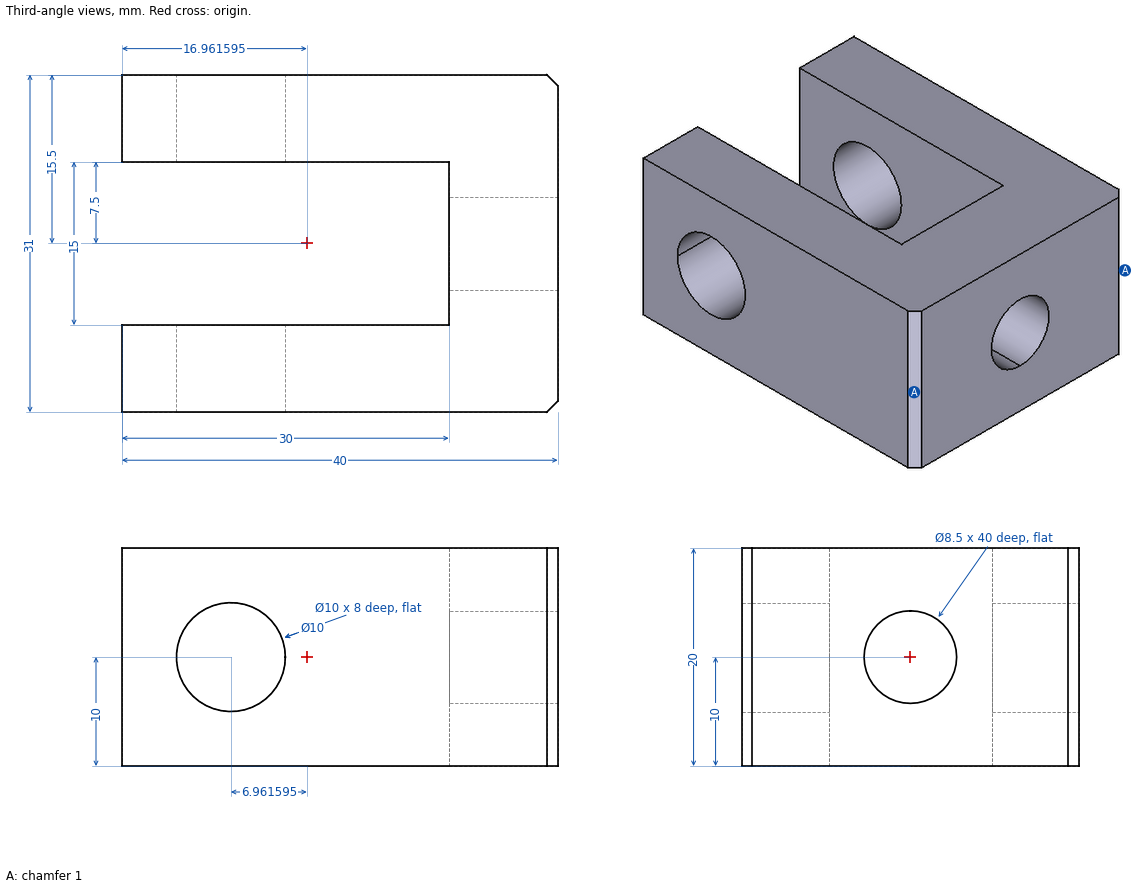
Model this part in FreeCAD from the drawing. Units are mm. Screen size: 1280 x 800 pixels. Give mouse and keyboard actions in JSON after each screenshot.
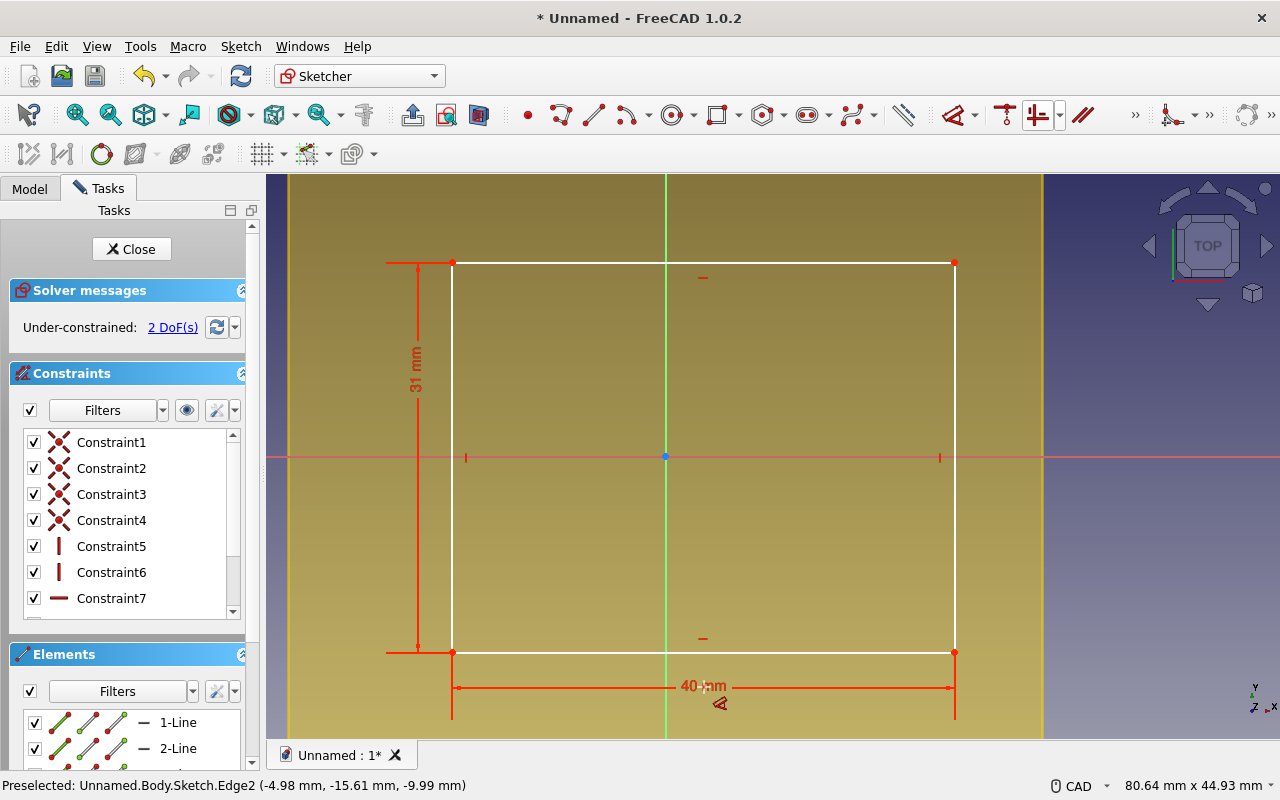
{"action": "left_click", "coordinate": [452, 263]}
{"action": "left_click", "coordinate": [418, 315]}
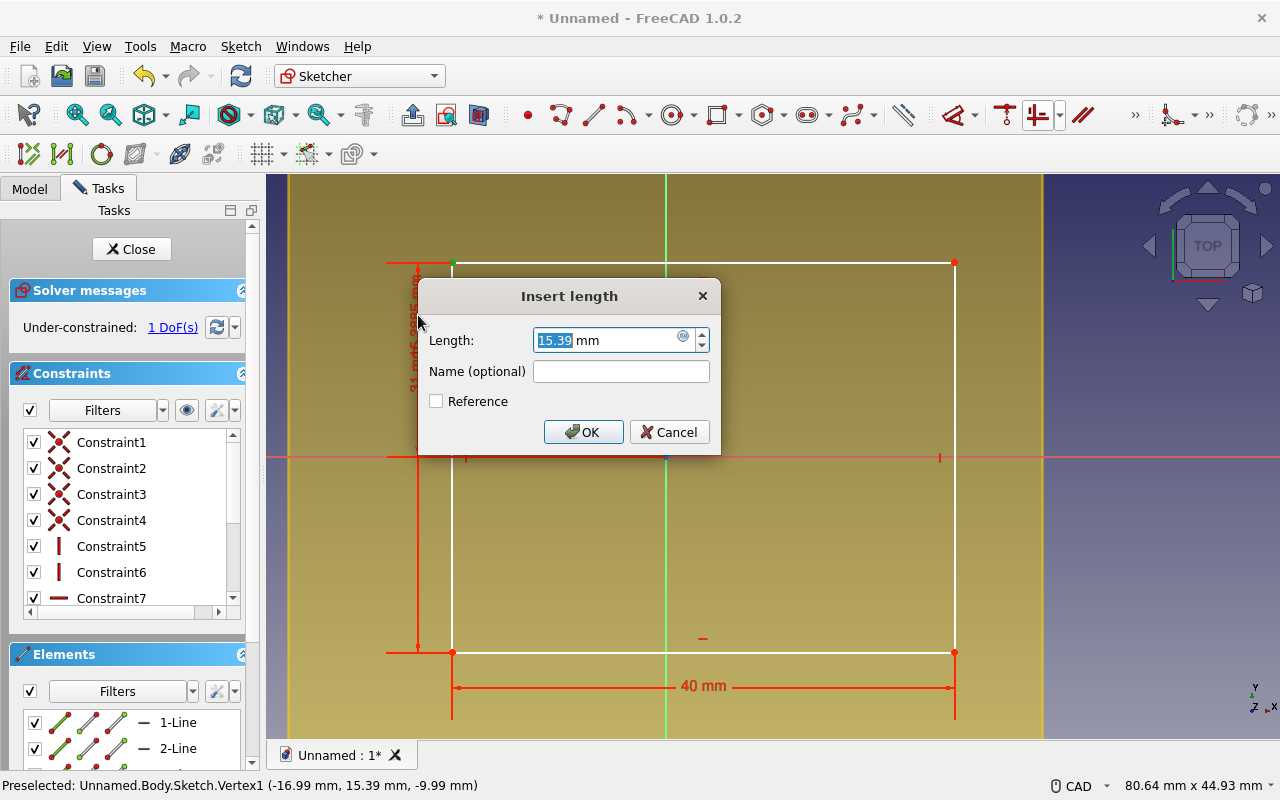
{"action": "type", "text": "15.5"}
{"action": "key", "text": "Return"}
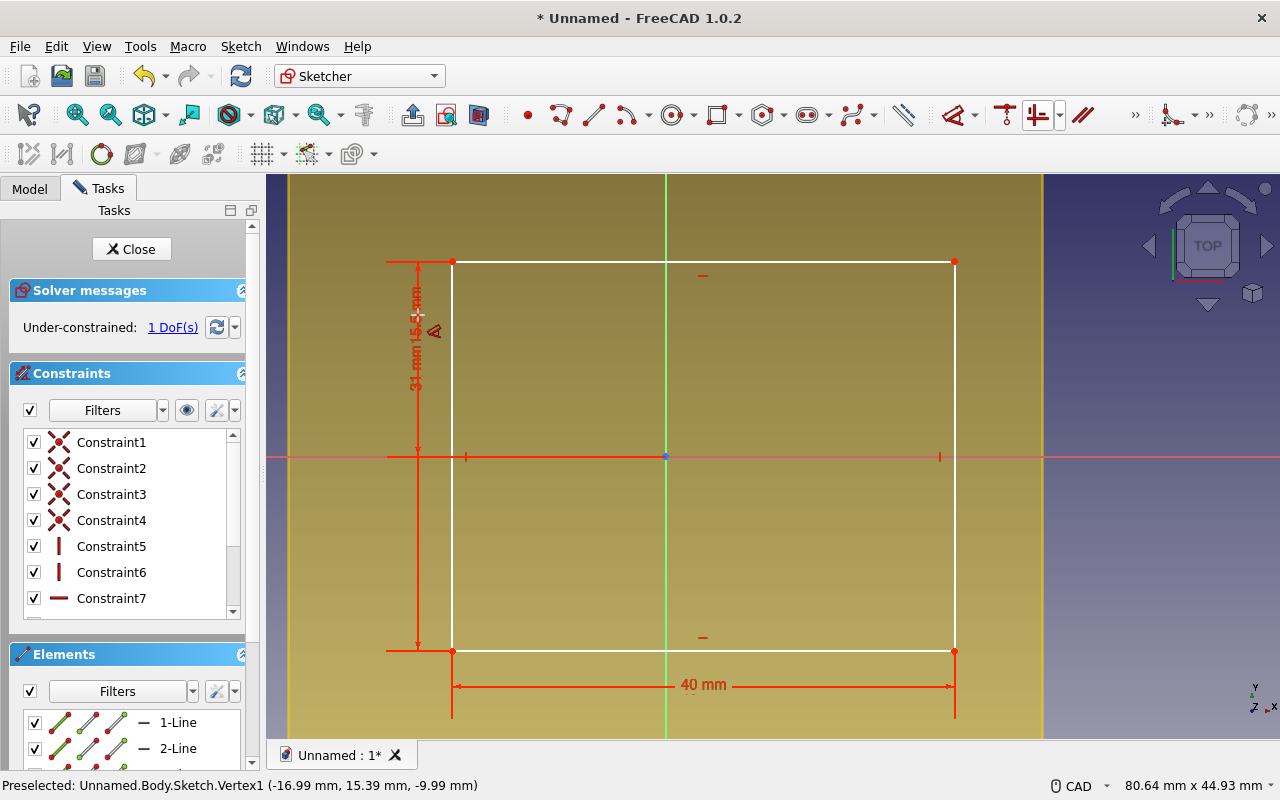
{"action": "left_click", "coordinate": [452, 262]}
{"action": "left_click", "coordinate": [559, 228]}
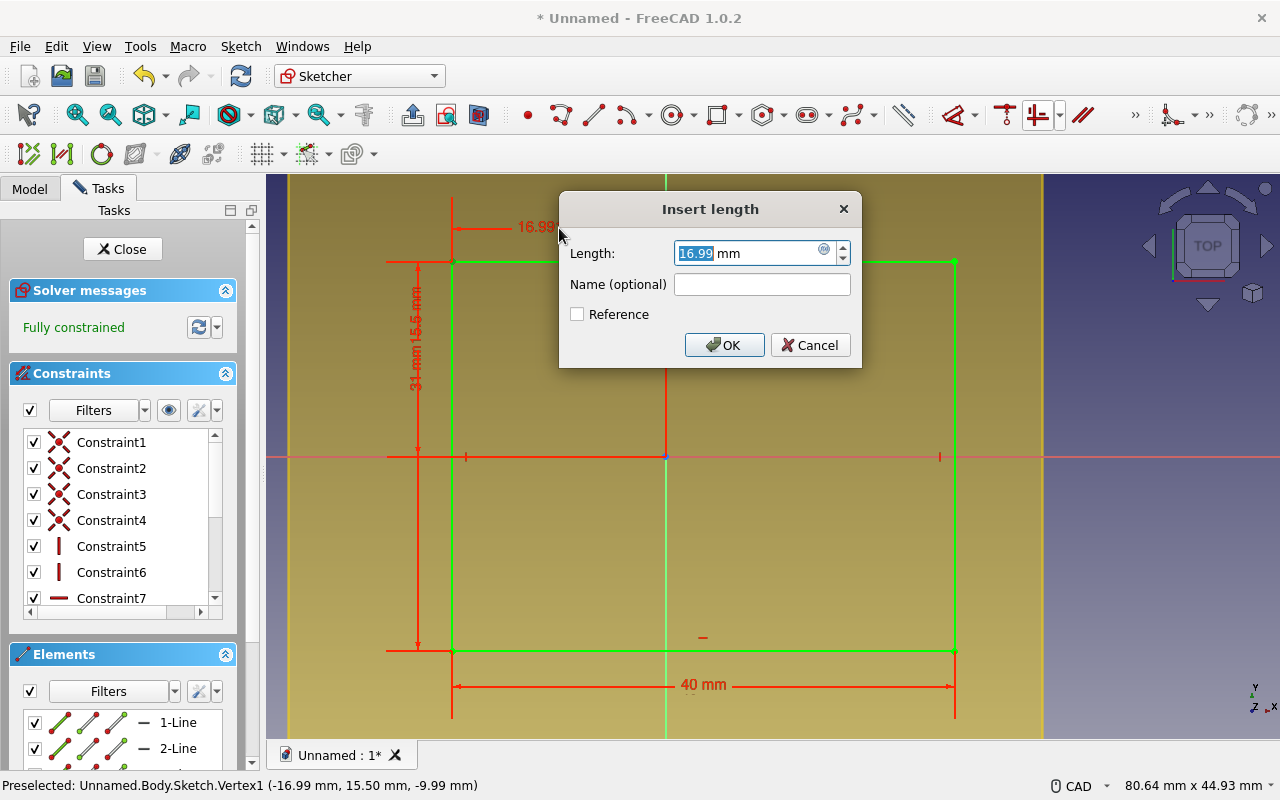
{"action": "type", "text": "16.961595"}
{"action": "key", "text": "Return"}
{"action": "key", "text": "Escape"}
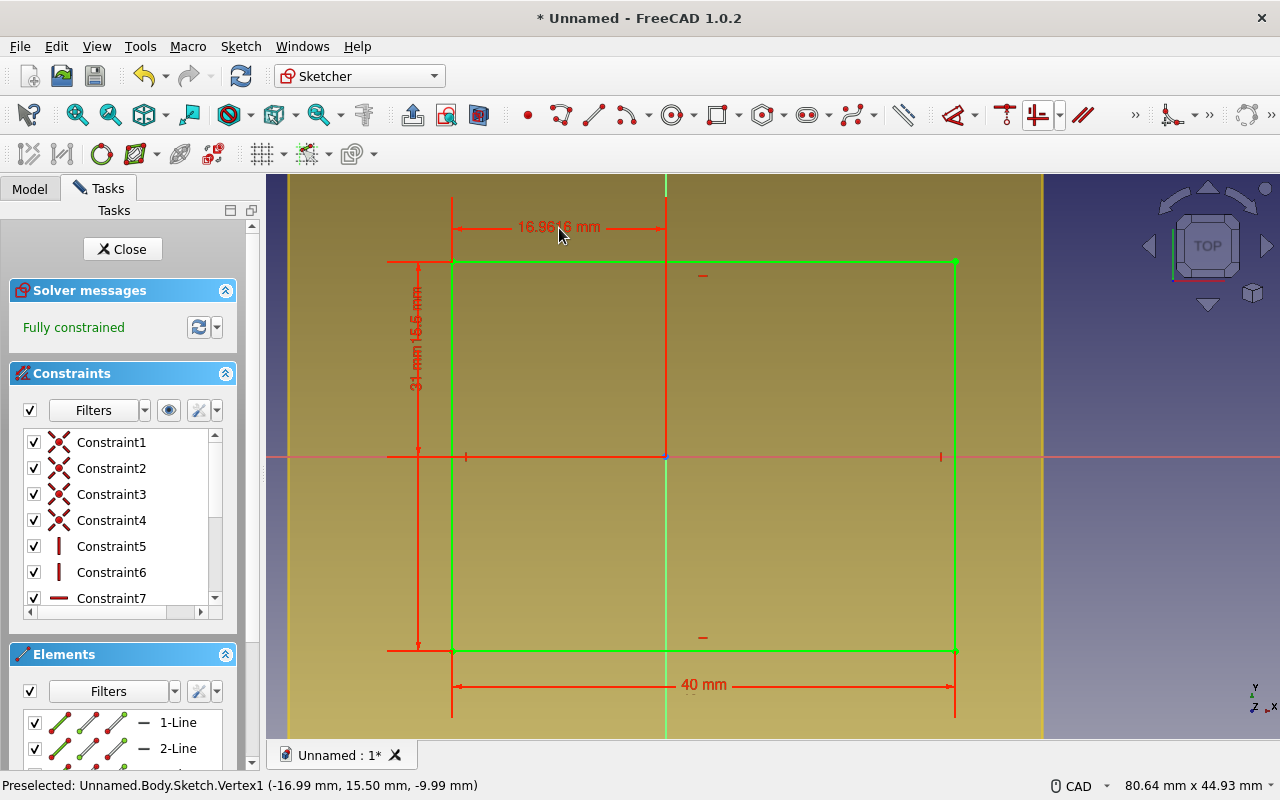
{"action": "left_click", "coordinate": [123, 249]}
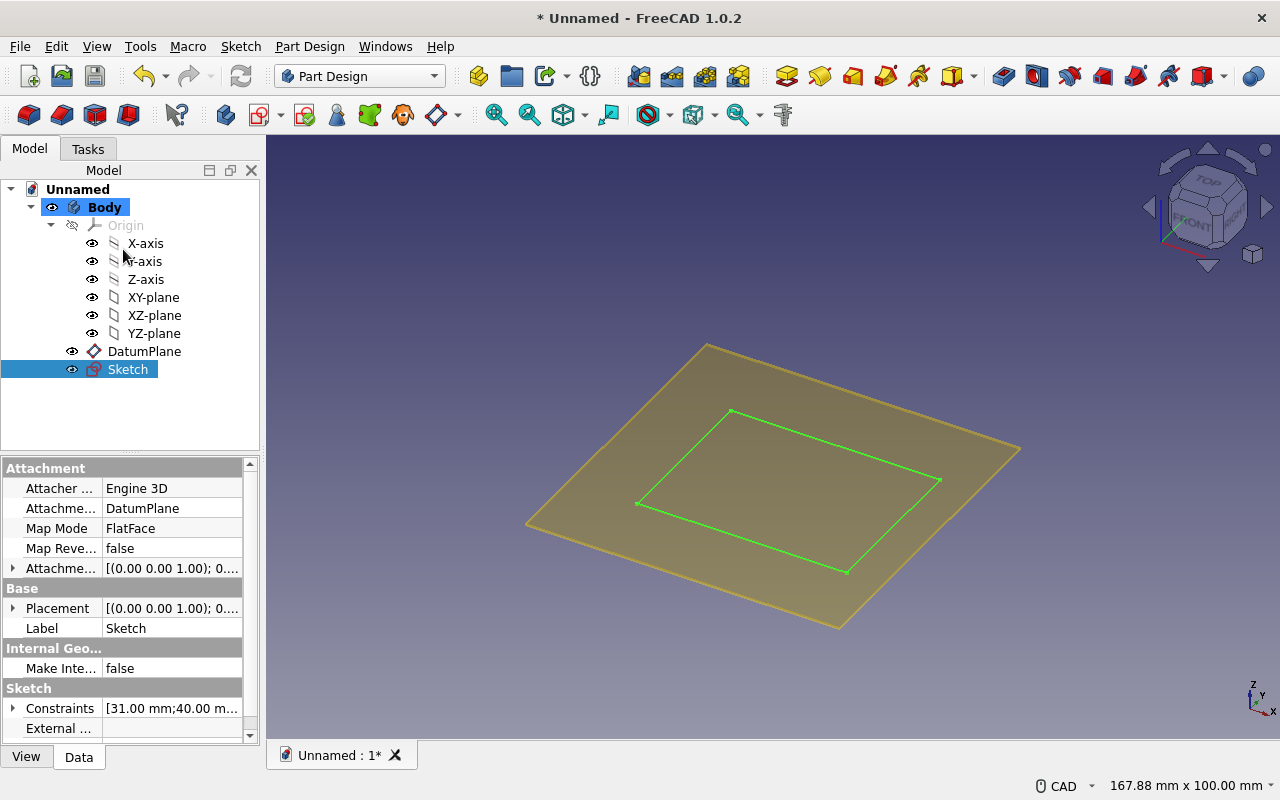
{"action": "left_click", "coordinate": [787, 76]}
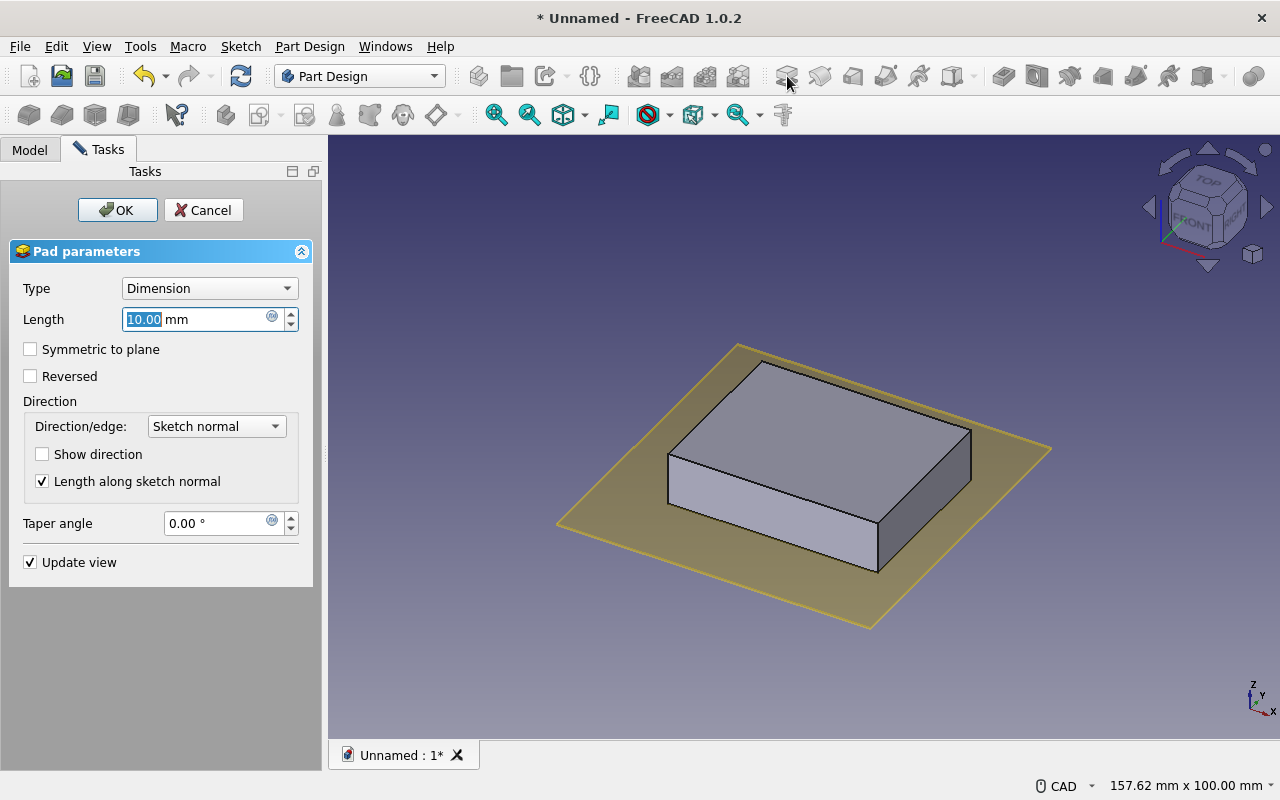
{"action": "type", "text": "20"}
{"action": "key", "text": "Tab"}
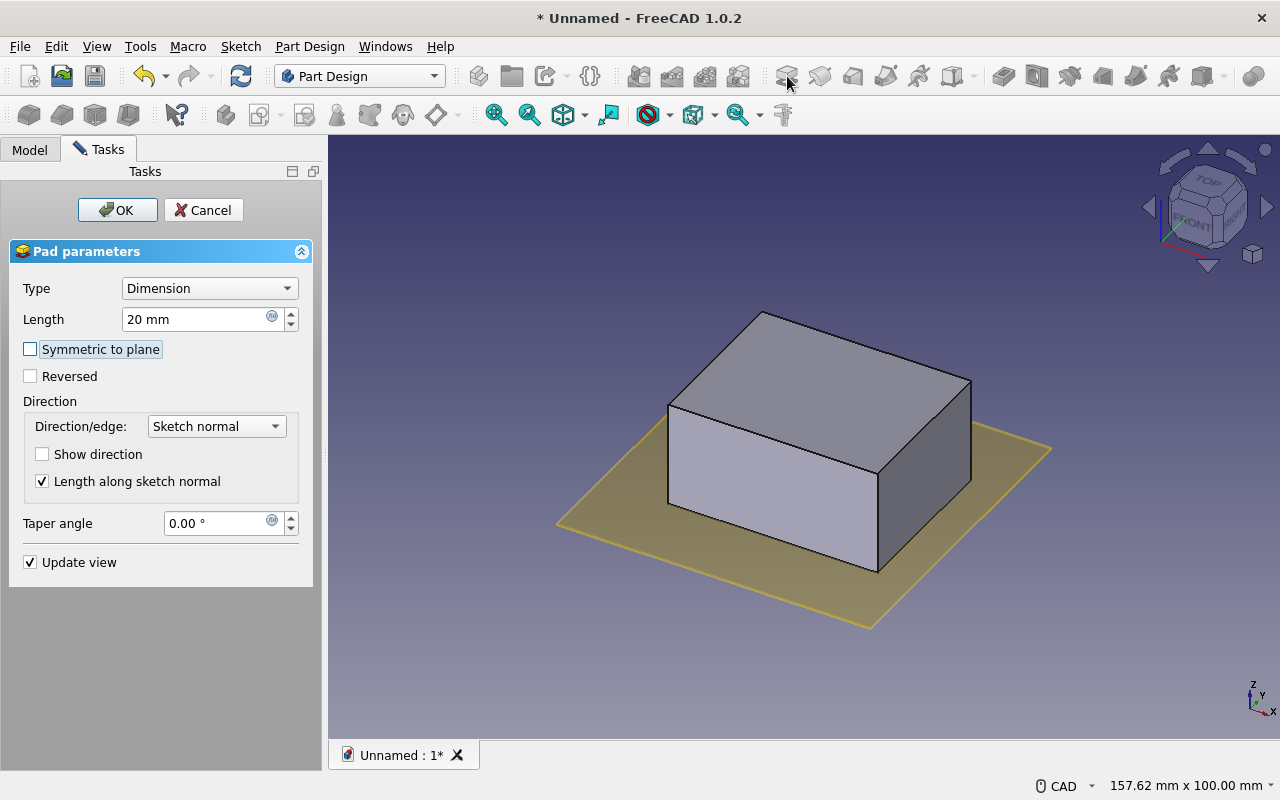
{"action": "left_click", "coordinate": [118, 210]}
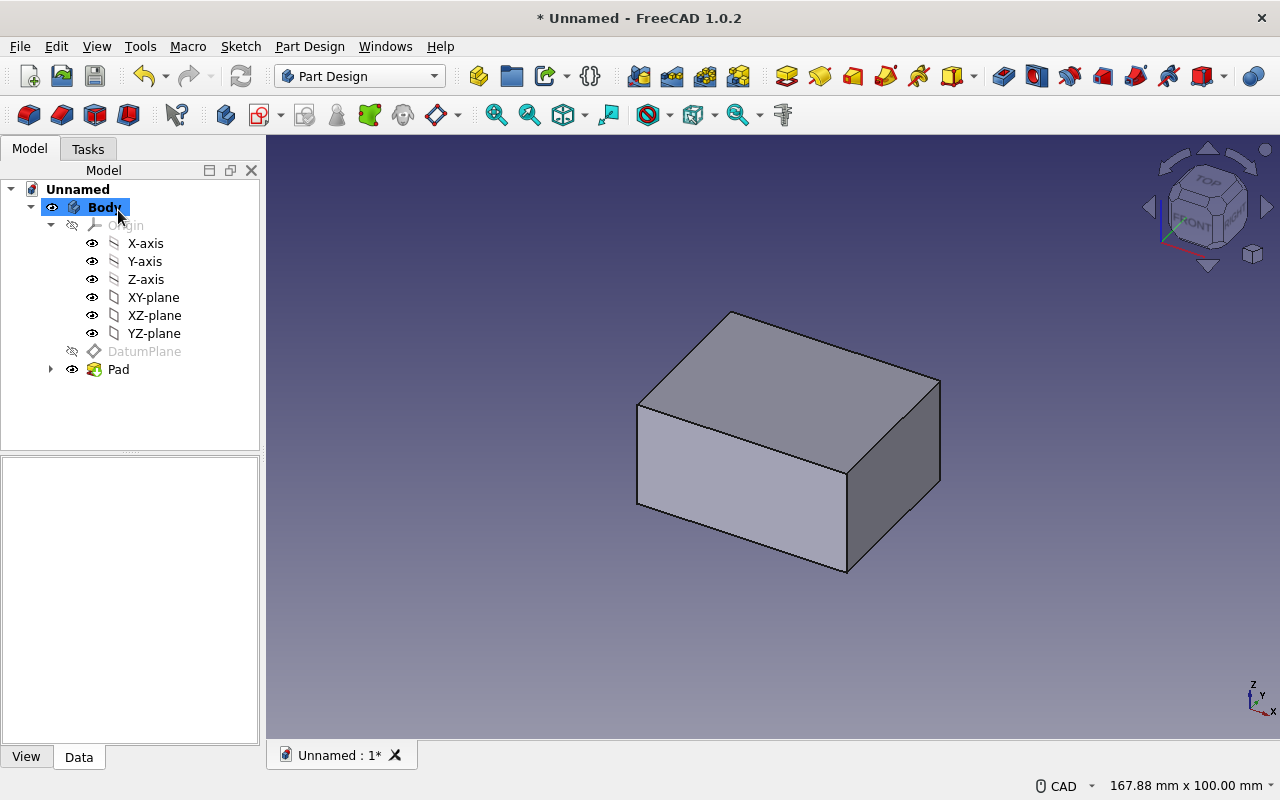
{"action": "left_click", "coordinate": [497, 116]}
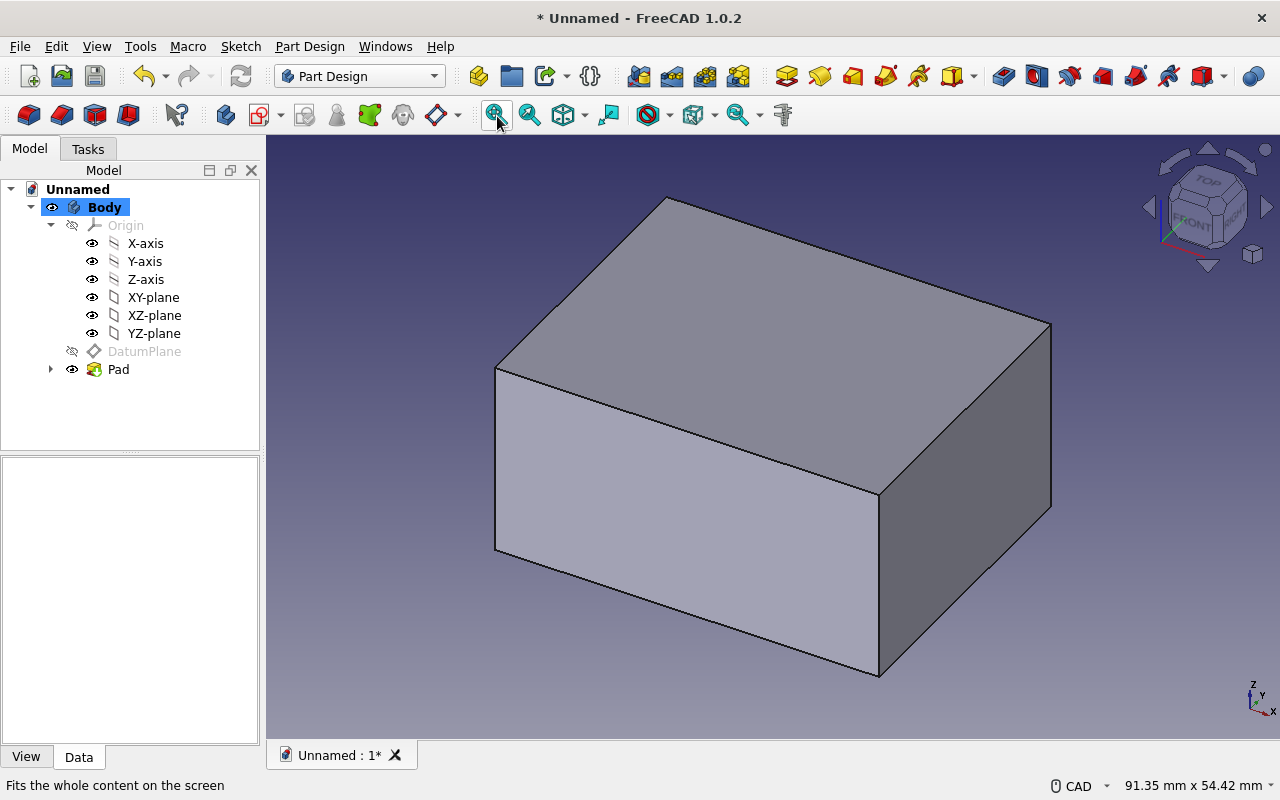
{"action": "left_click", "coordinate": [773, 345]}